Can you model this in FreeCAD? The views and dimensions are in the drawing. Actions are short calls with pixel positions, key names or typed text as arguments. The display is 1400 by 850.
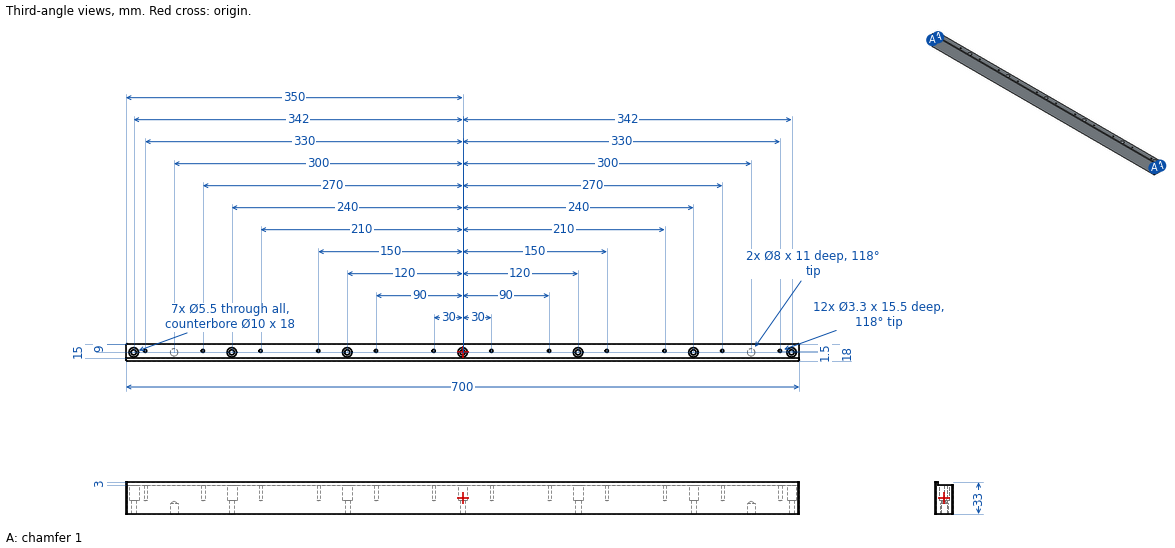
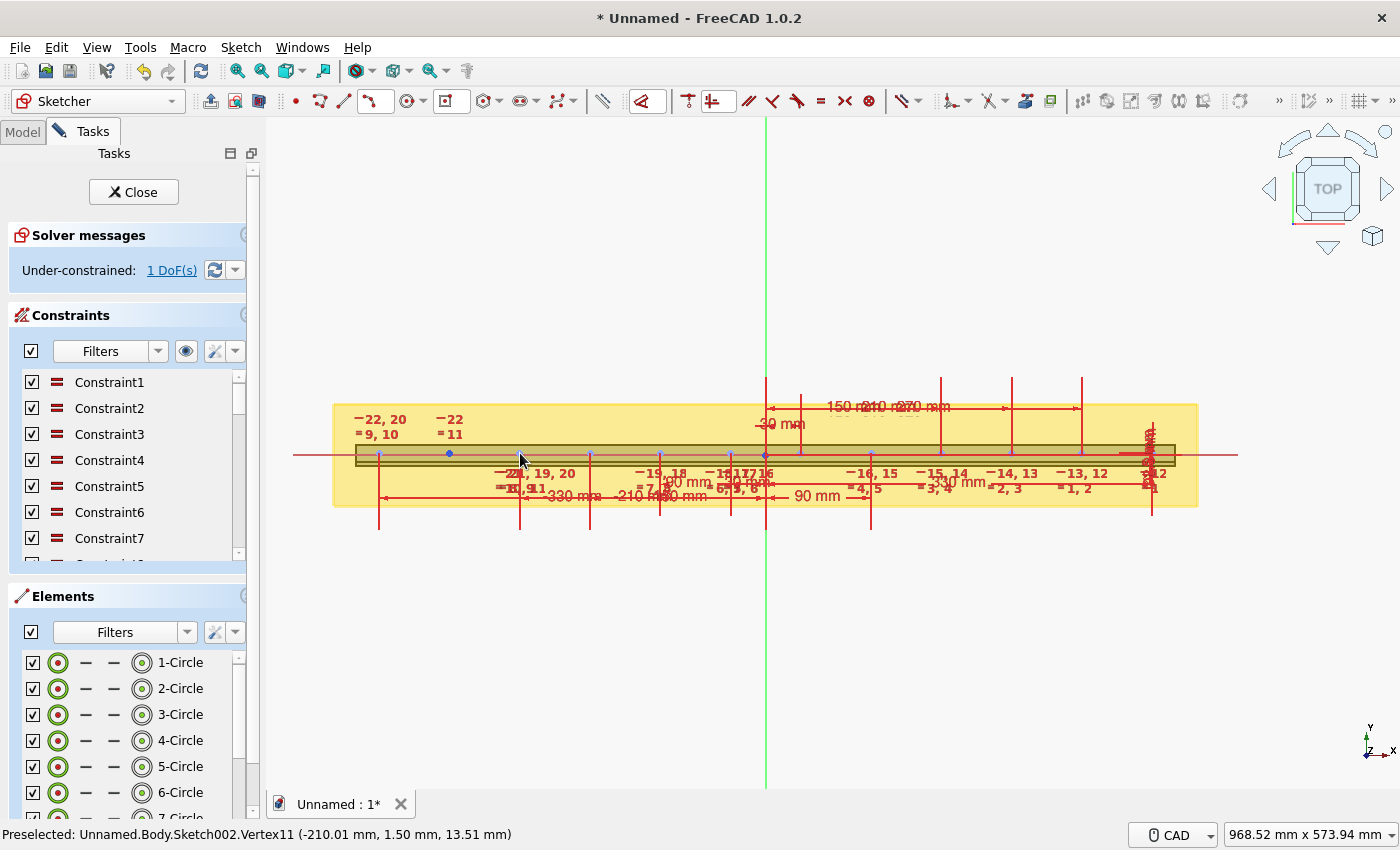
click(449, 453)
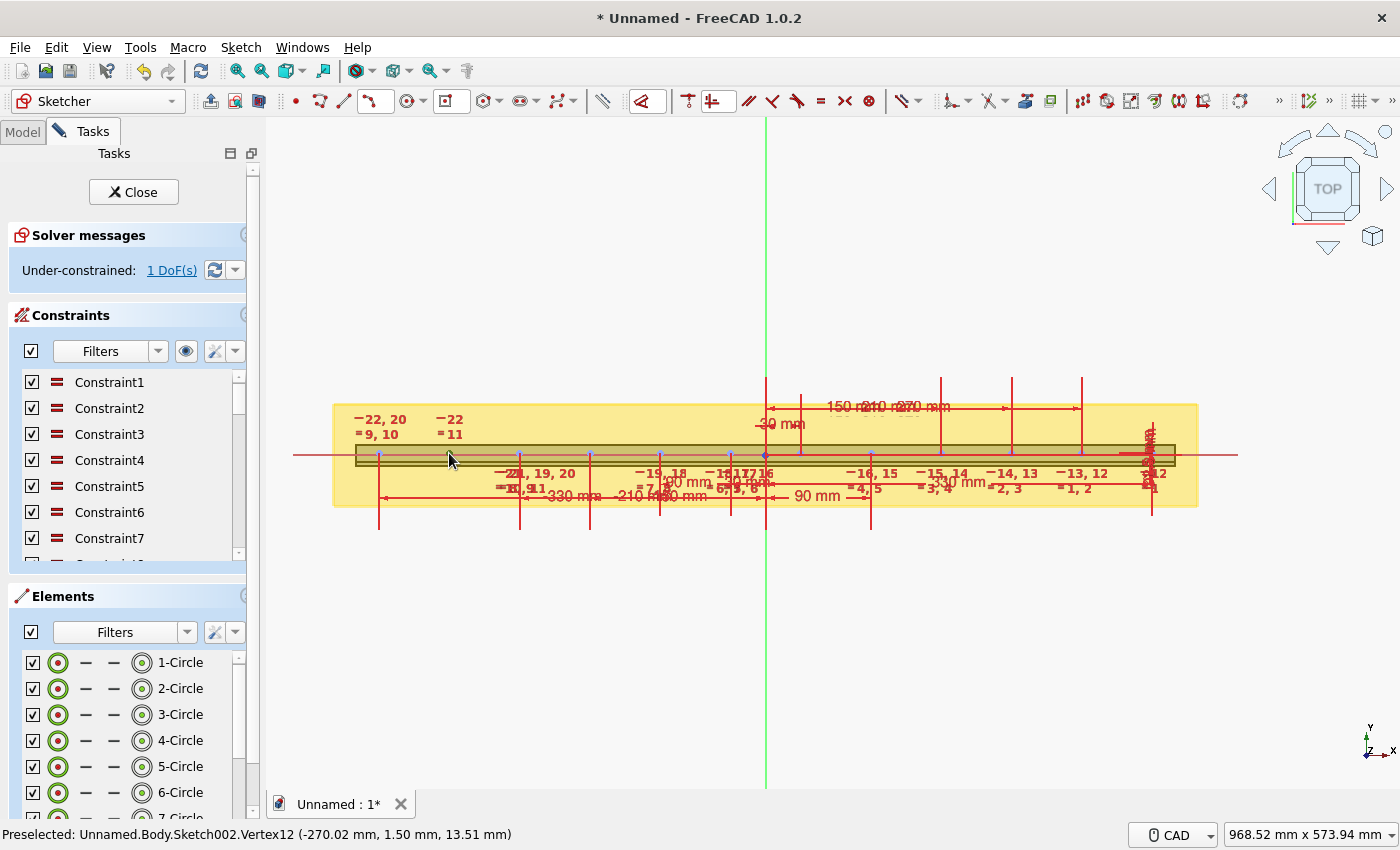
key(l)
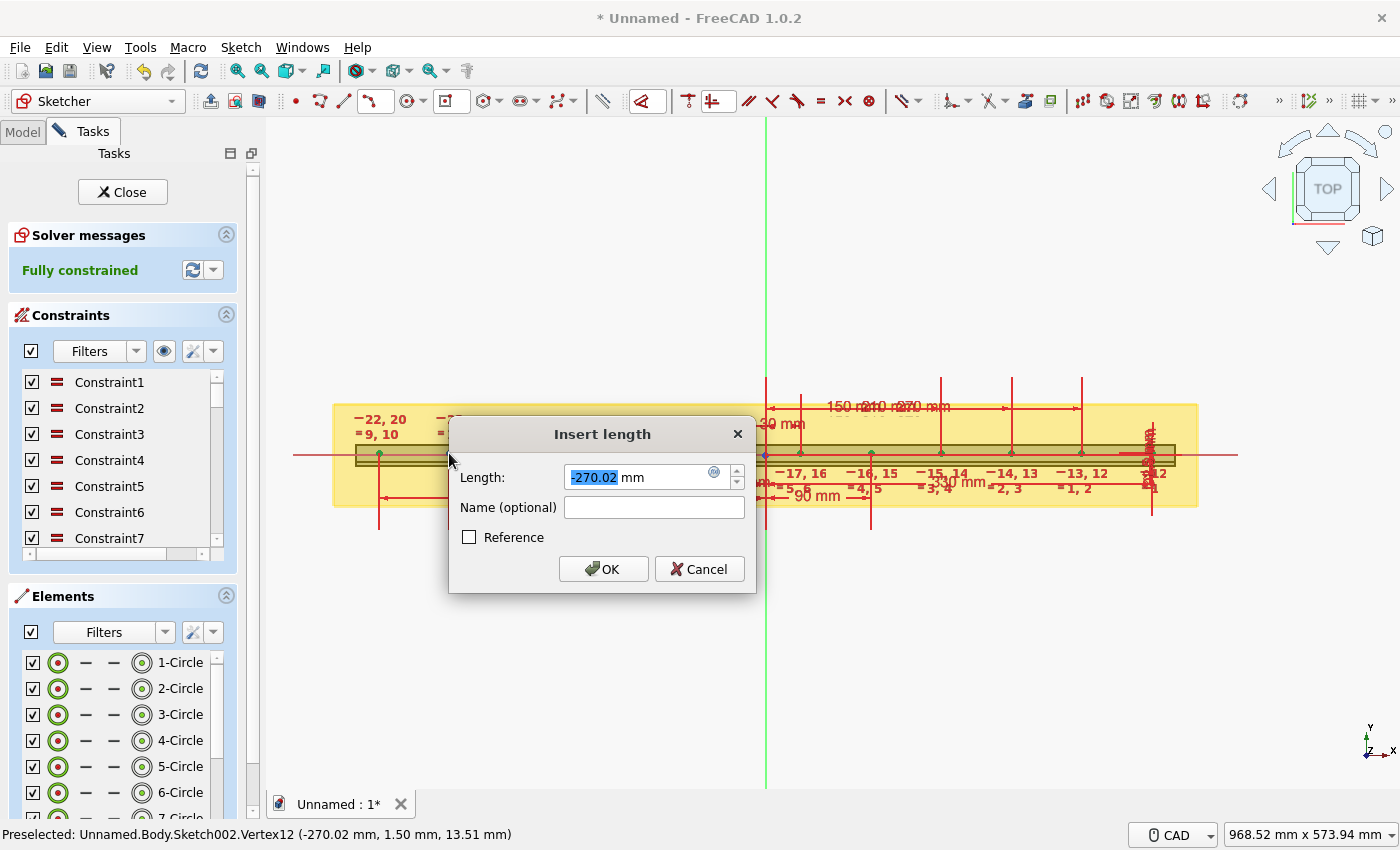
text(-270)
key(Return)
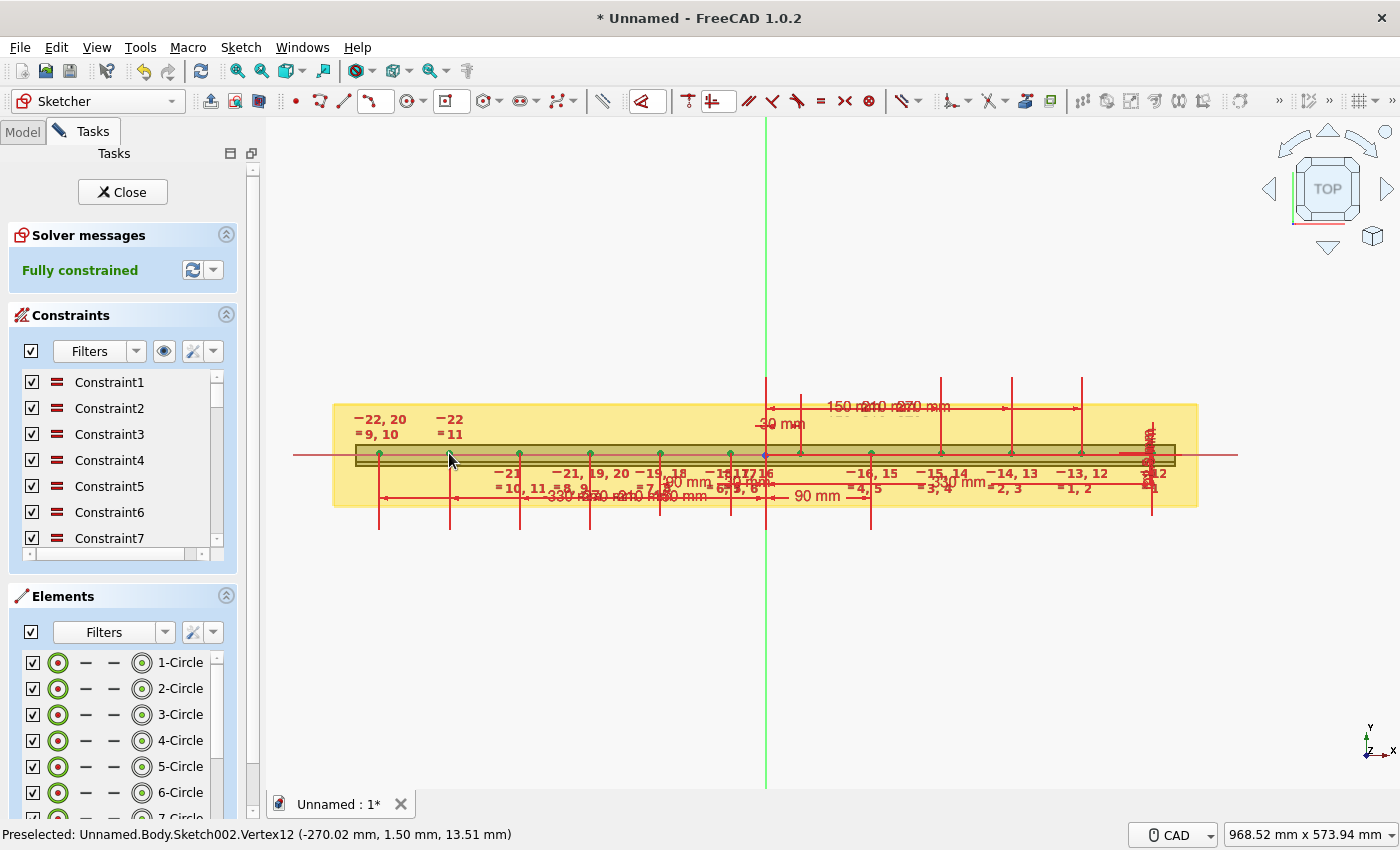
click(123, 192)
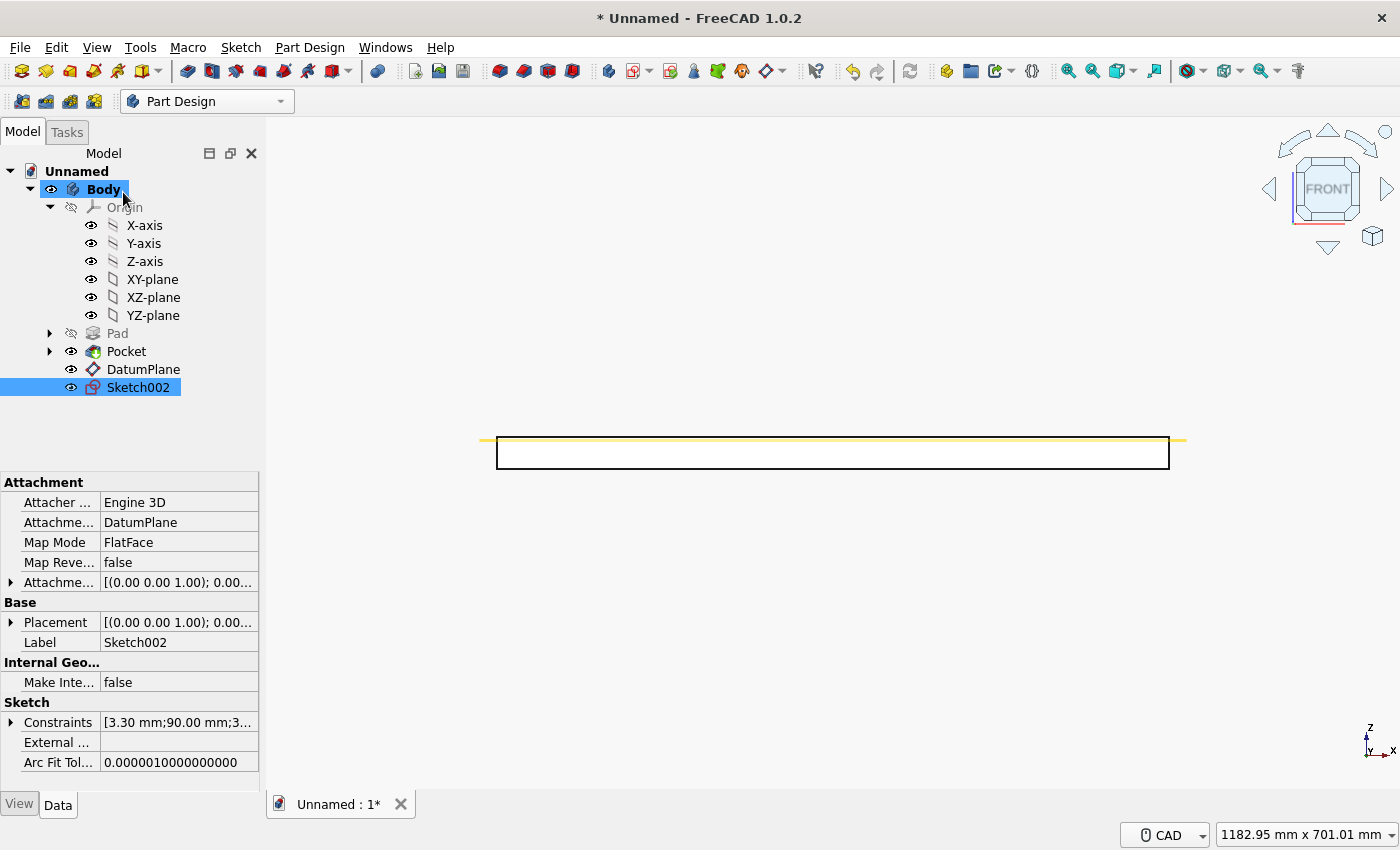
click(212, 72)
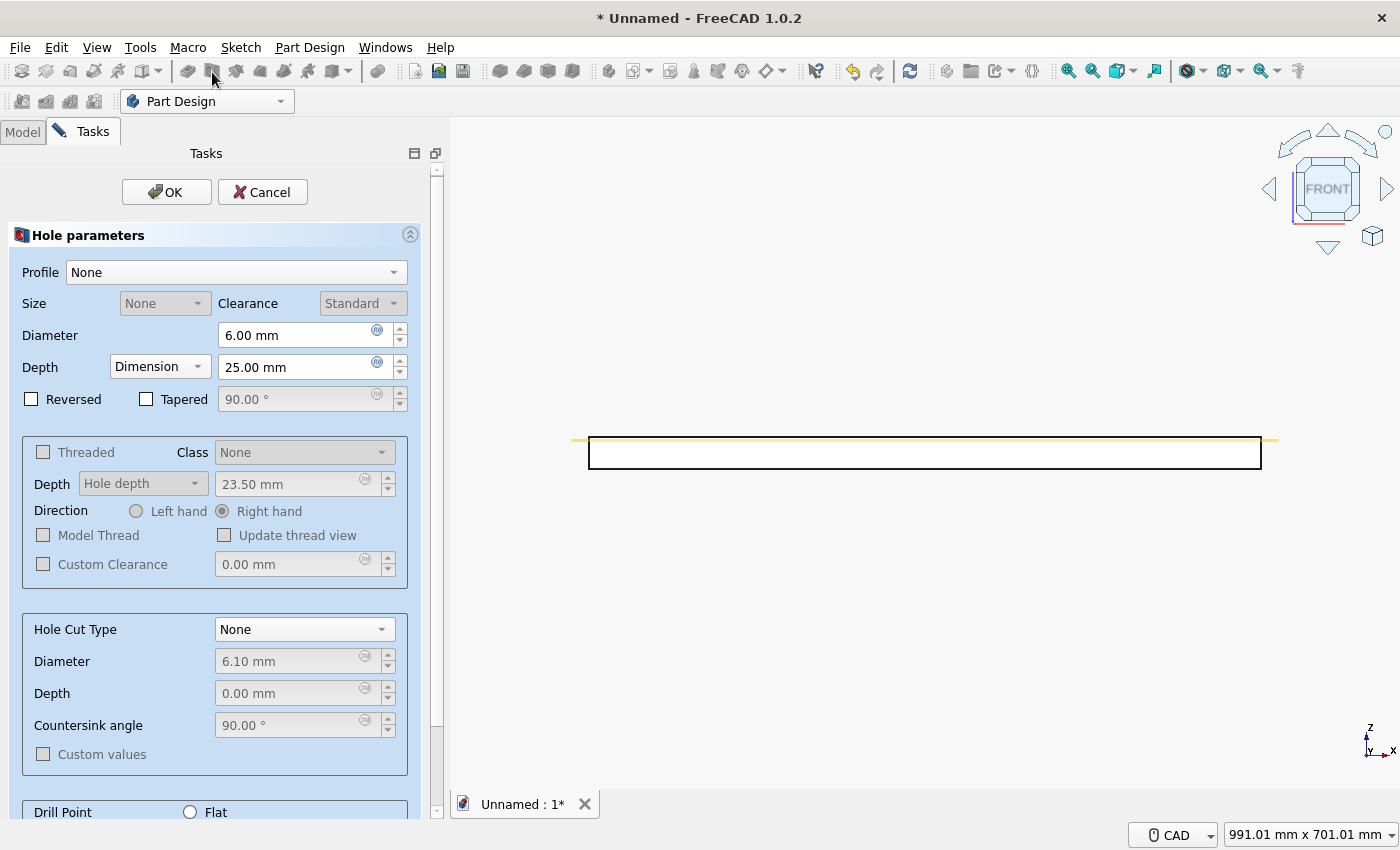
triple_click(305, 335)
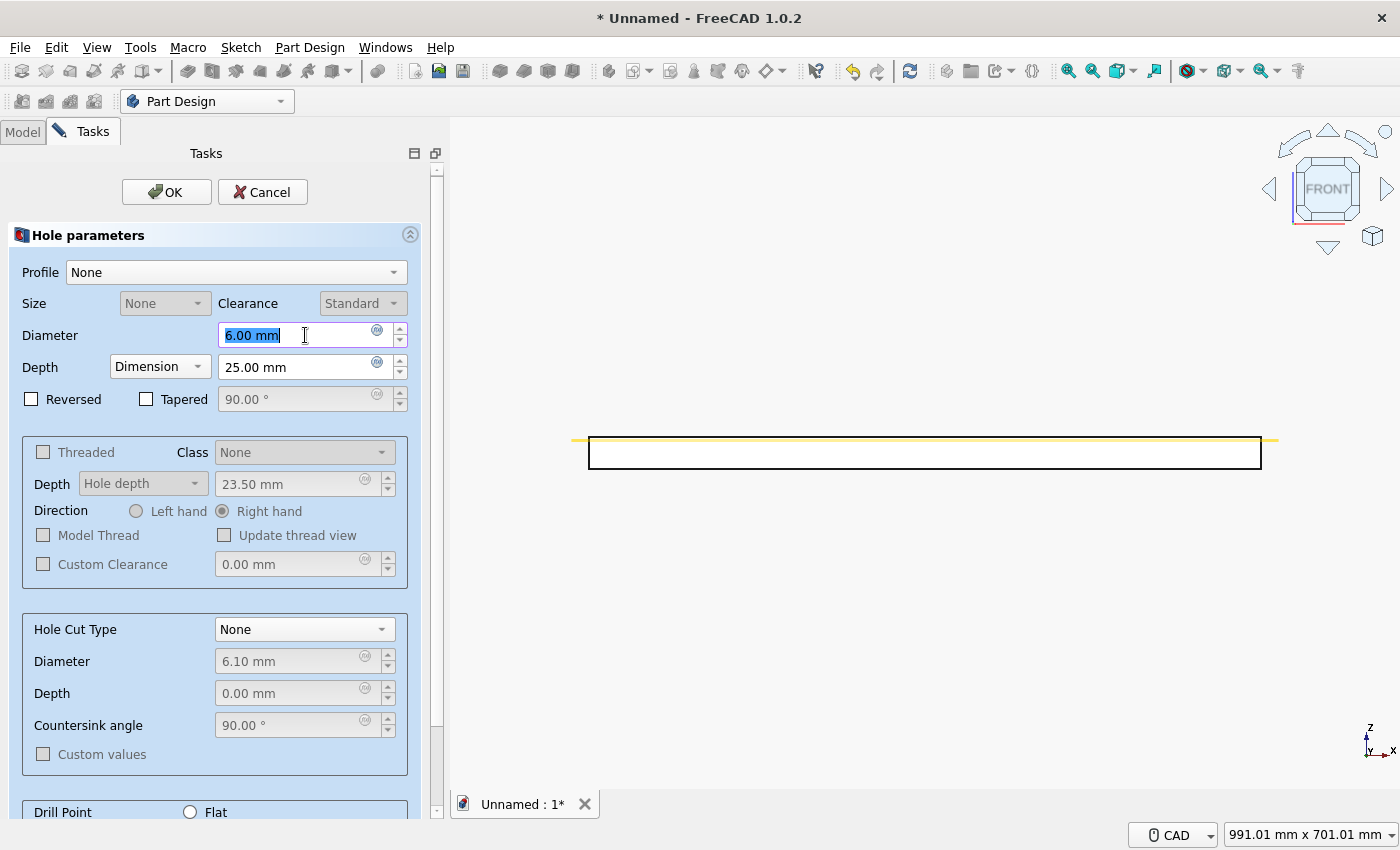
text(3.3)
key(Tab)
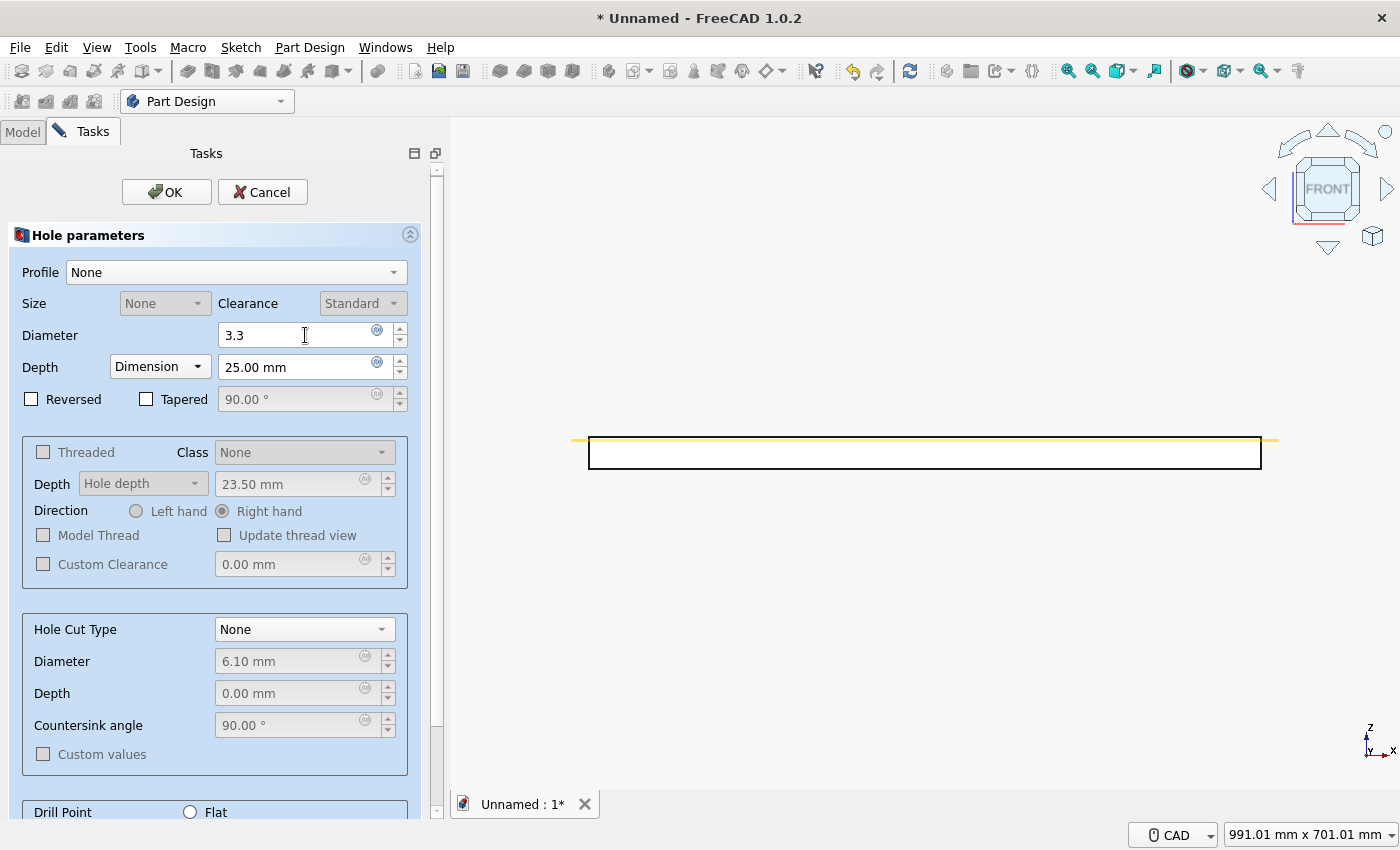
triple_click(305, 367)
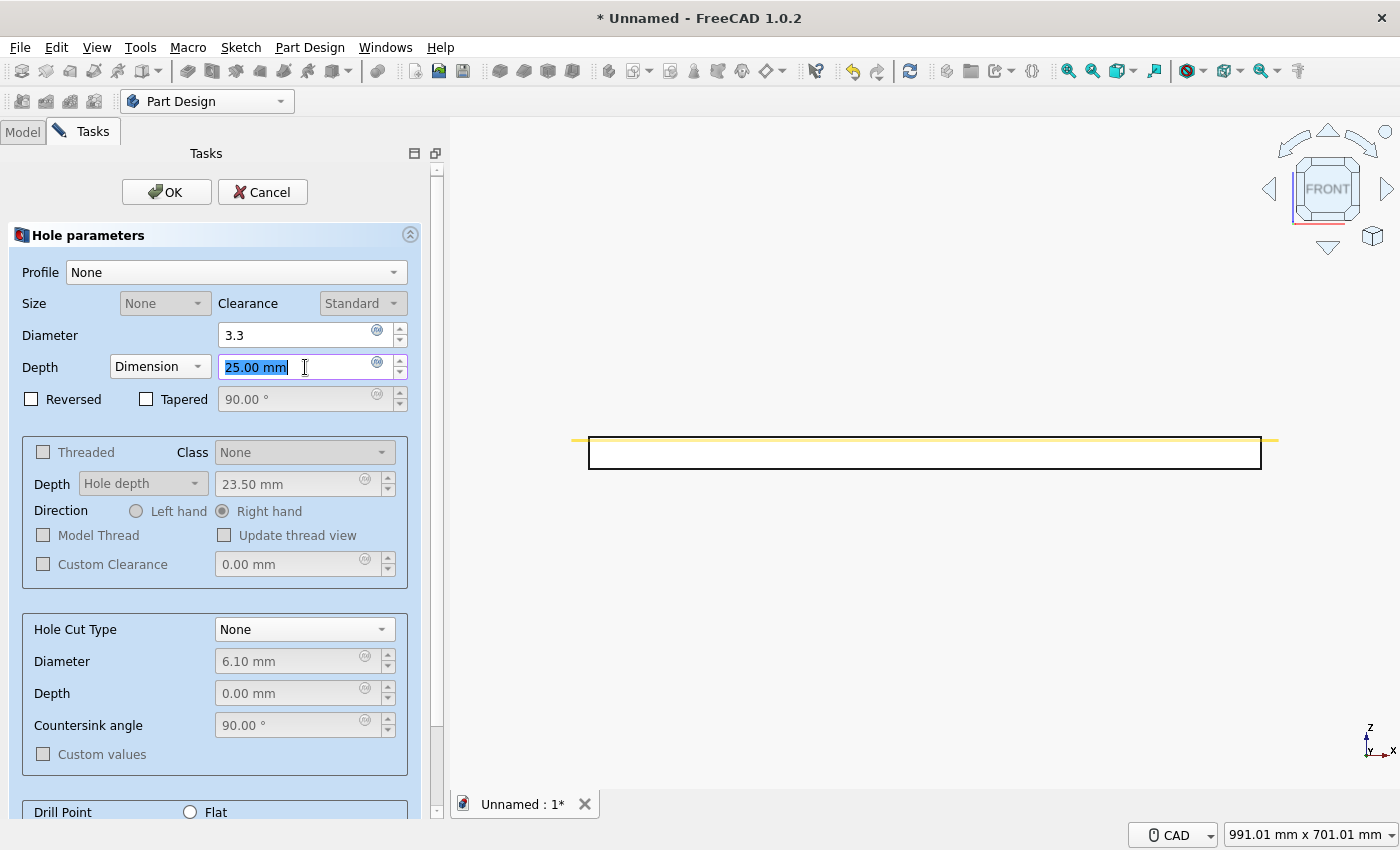
text(15.5)
key(Tab)